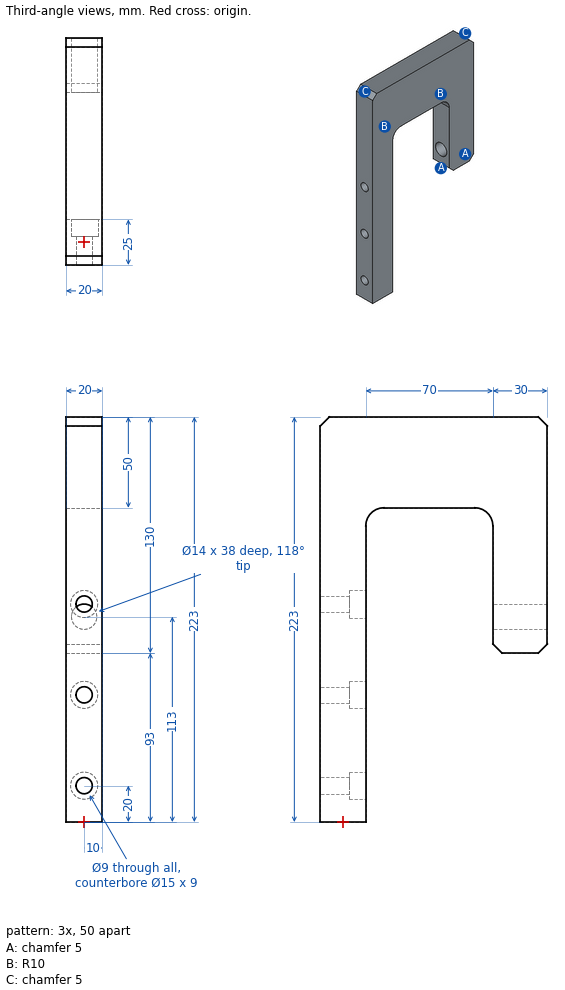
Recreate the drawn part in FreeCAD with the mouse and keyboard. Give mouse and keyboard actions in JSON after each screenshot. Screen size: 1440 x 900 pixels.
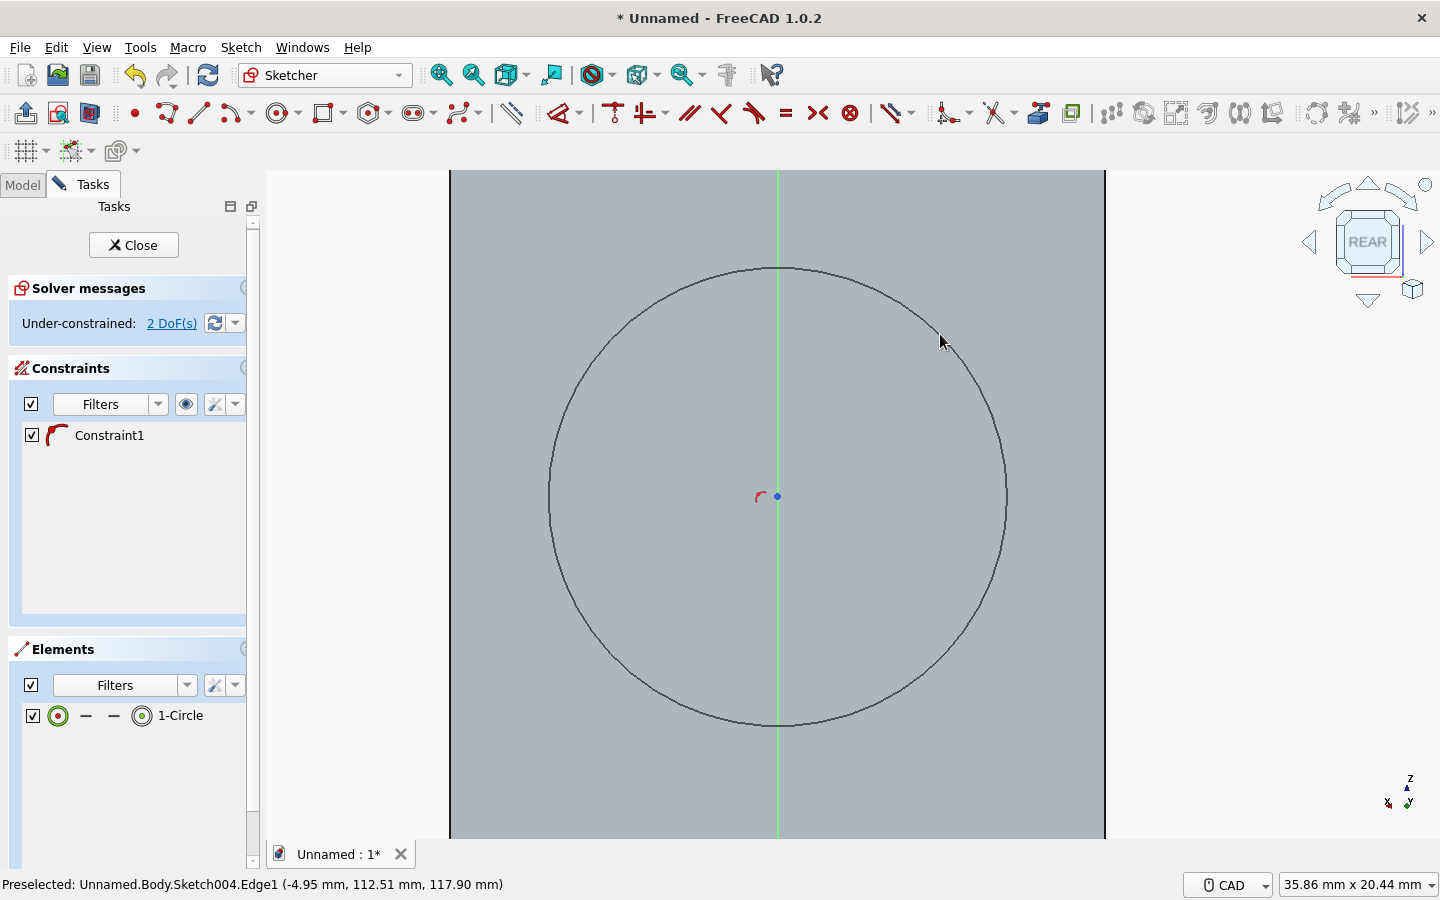
{"action": "left_click", "coordinate": [558, 114]}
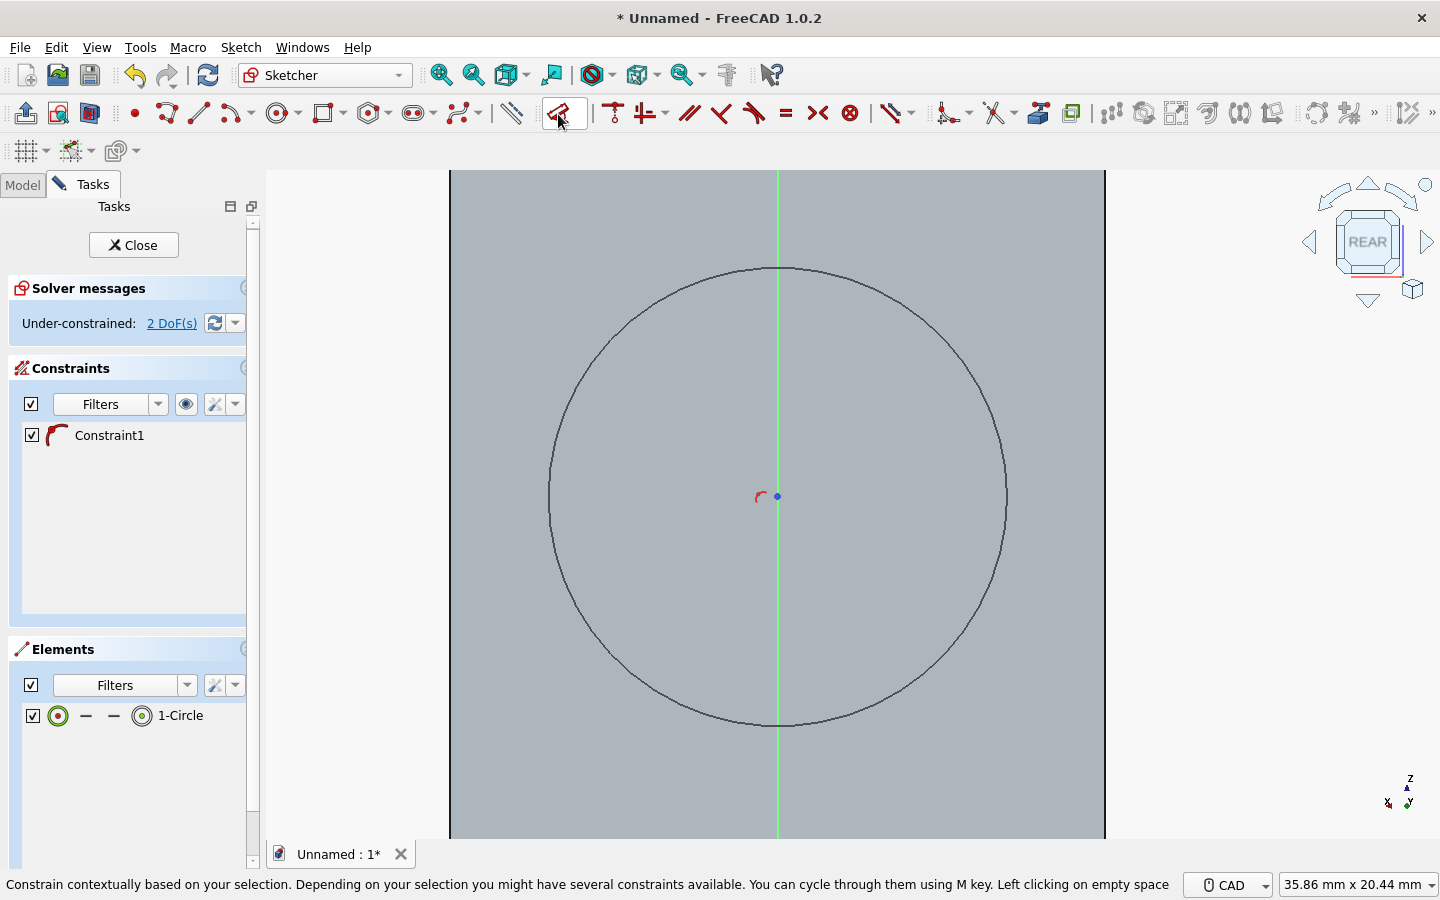
{"action": "left_click", "coordinate": [939, 334]}
{"action": "left_click", "coordinate": [962, 311]}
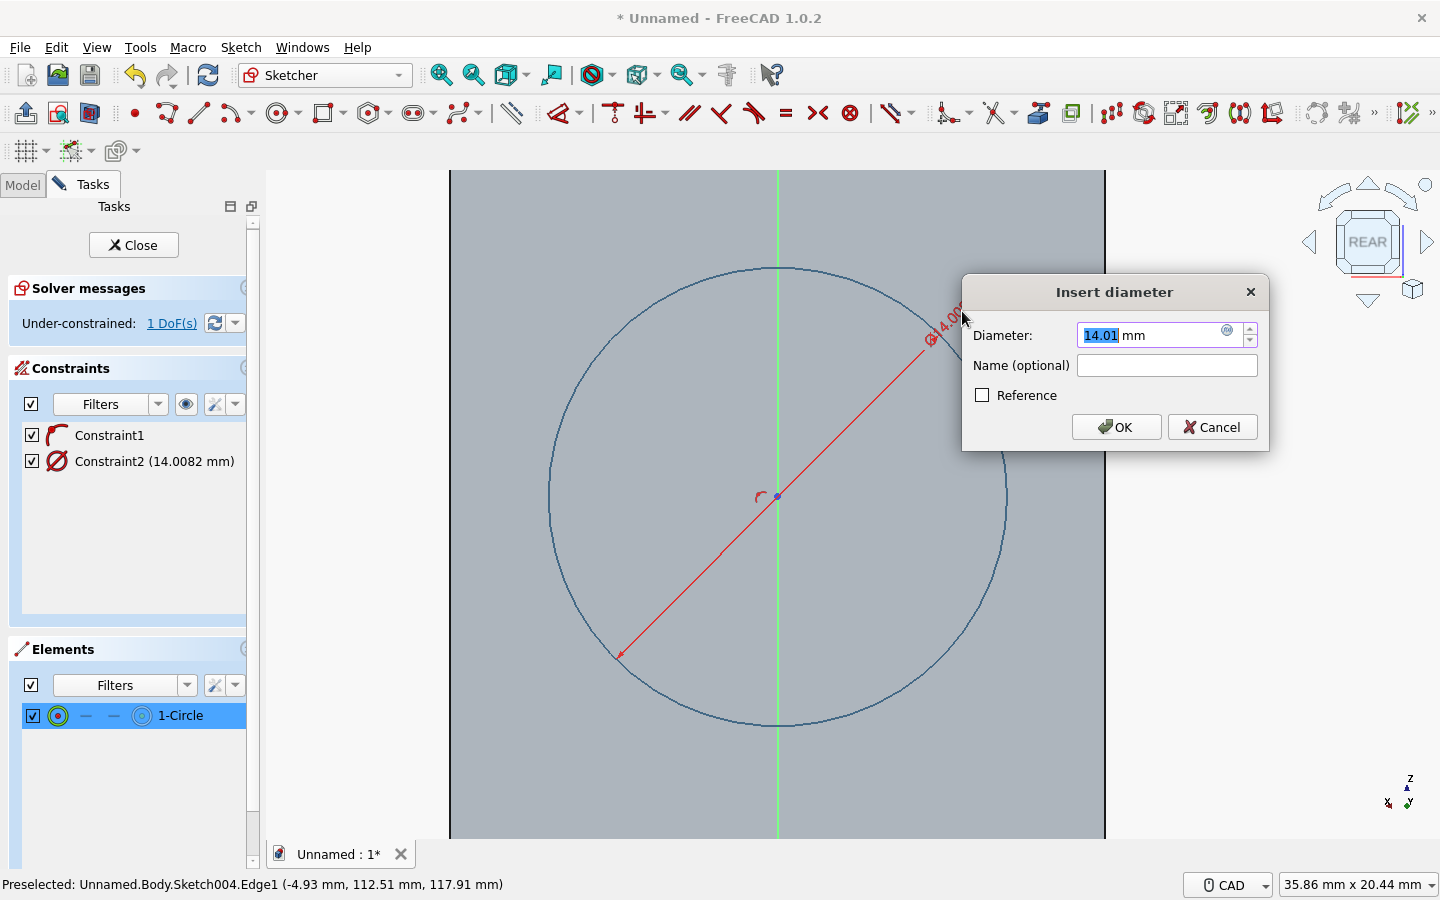
{"action": "type", "text": "14"}
{"action": "key", "text": "Return"}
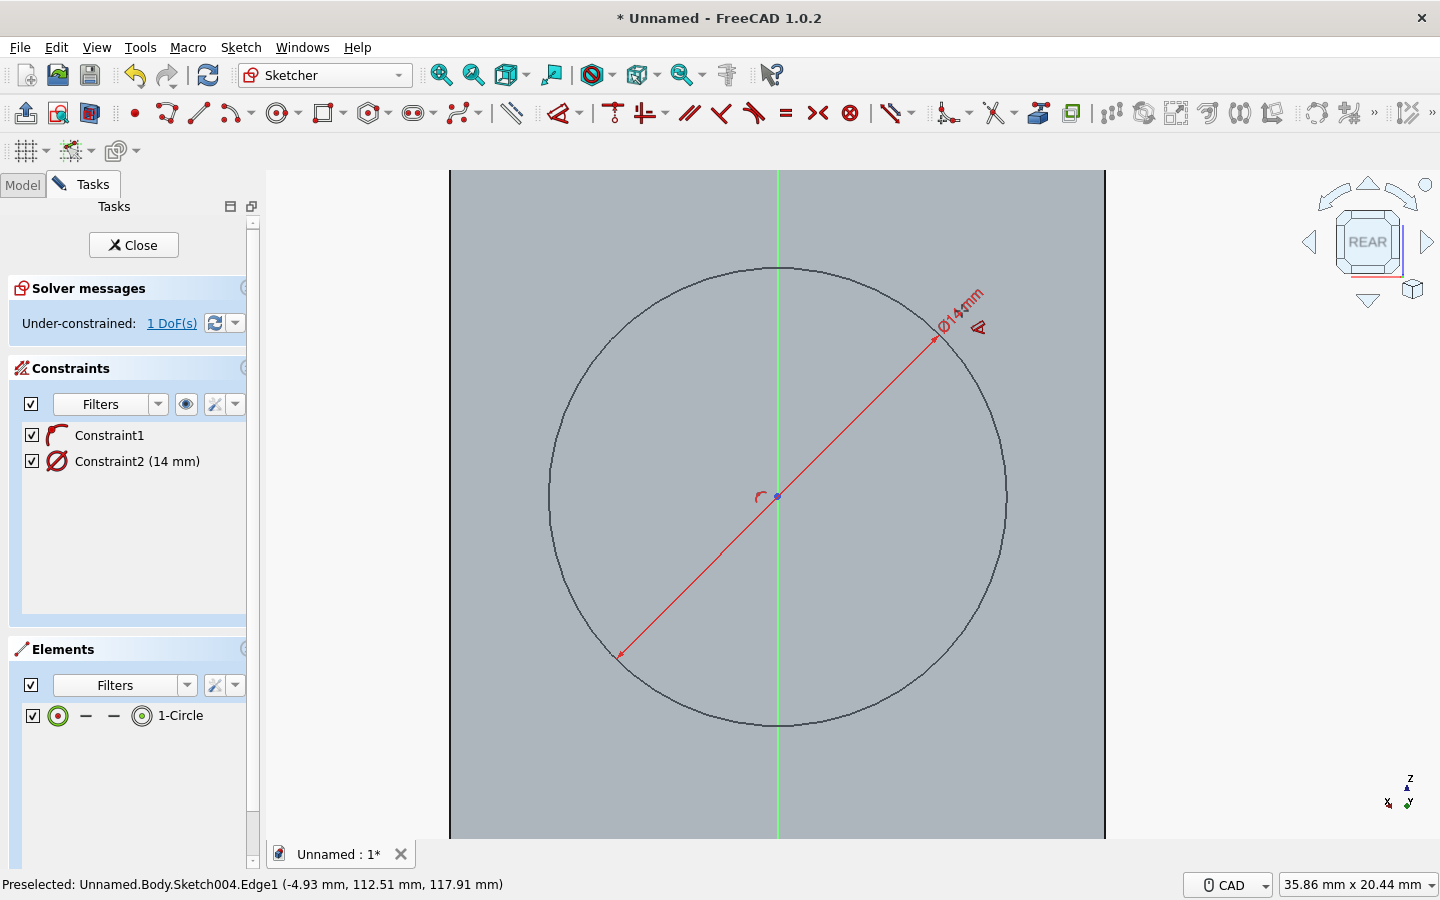
{"action": "left_click", "coordinate": [778, 497]}
{"action": "left_click", "coordinate": [812, 654]}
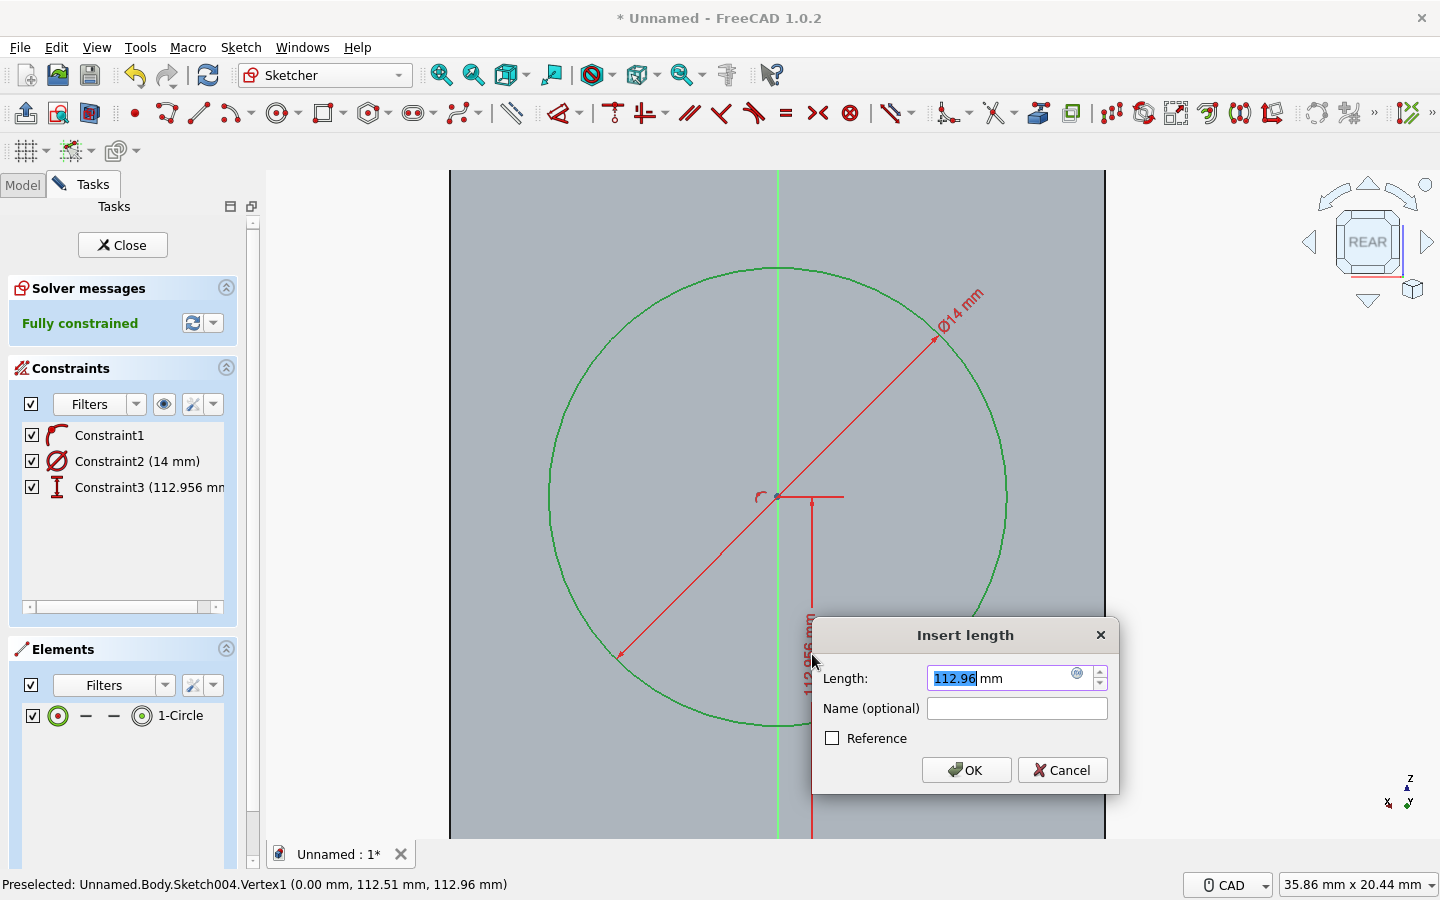
{"action": "type", "text": "113"}
{"action": "key", "text": "Return"}
{"action": "key", "text": "Escape"}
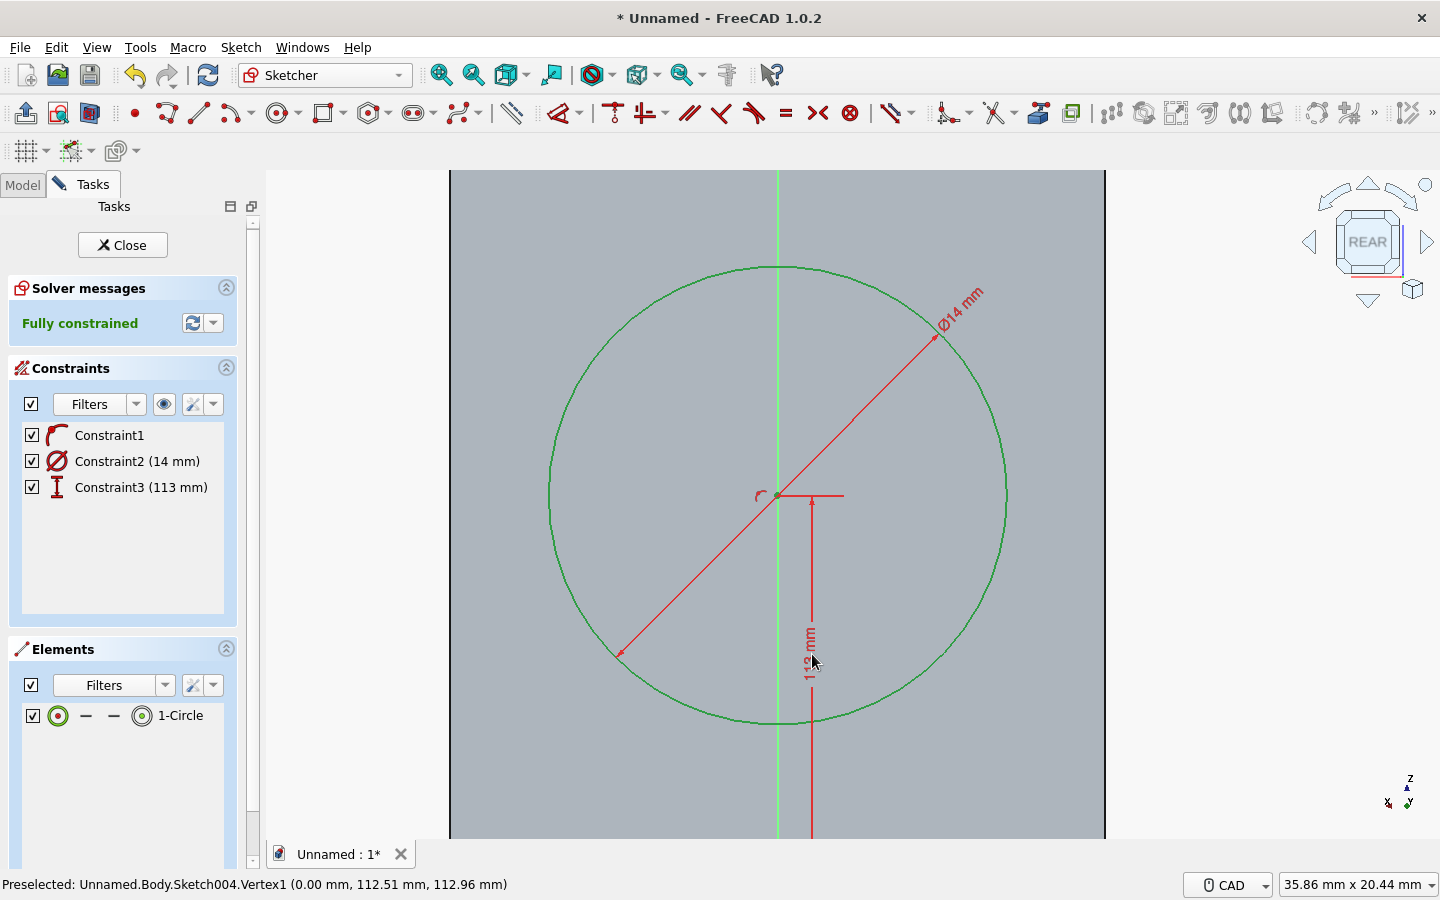
{"action": "left_click", "coordinate": [123, 245]}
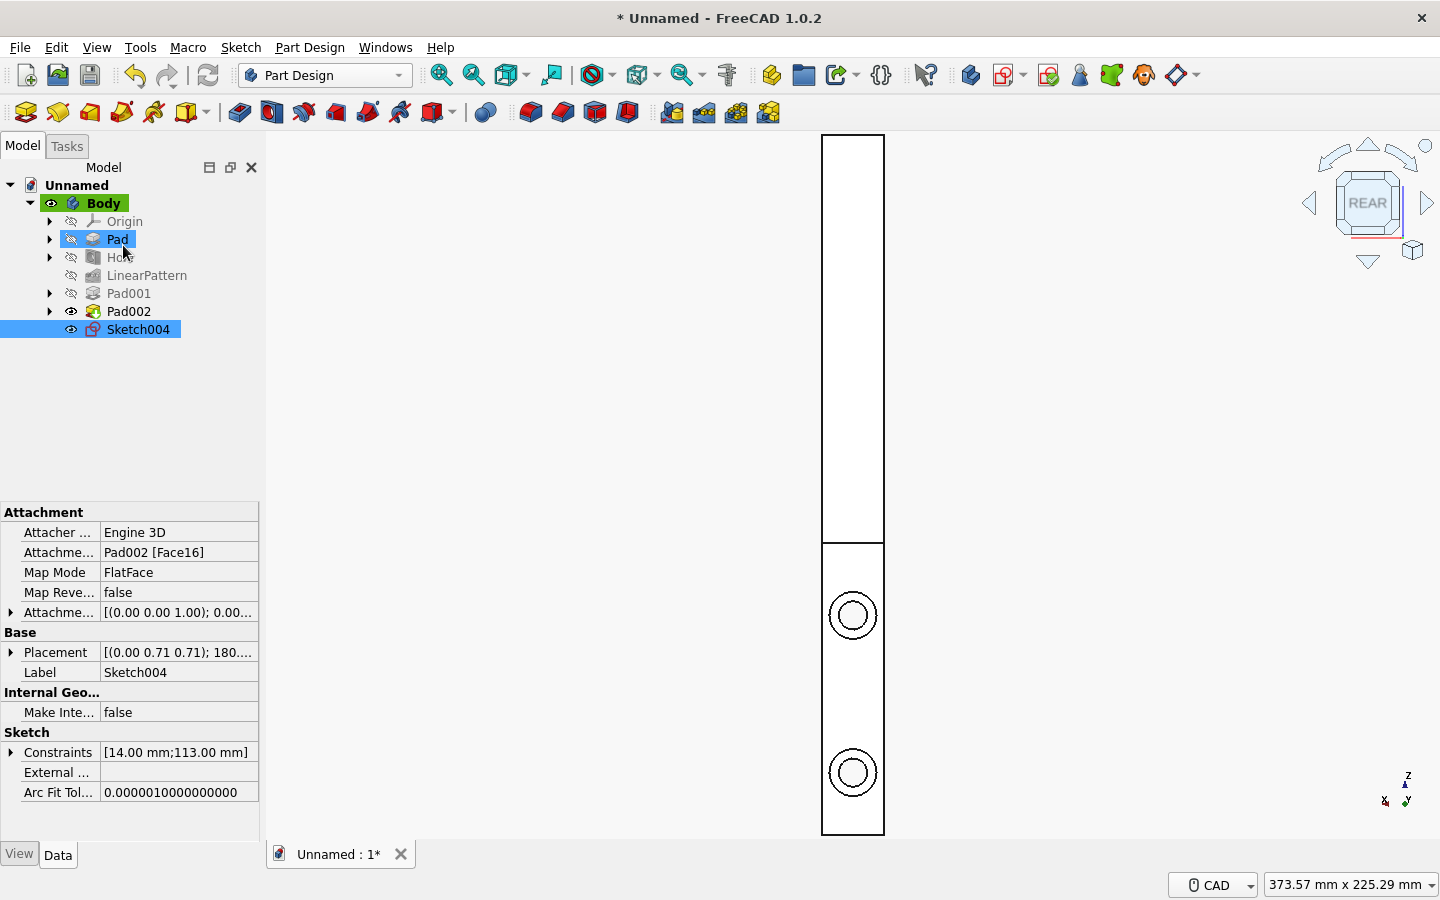
{"action": "left_click", "coordinate": [272, 112]}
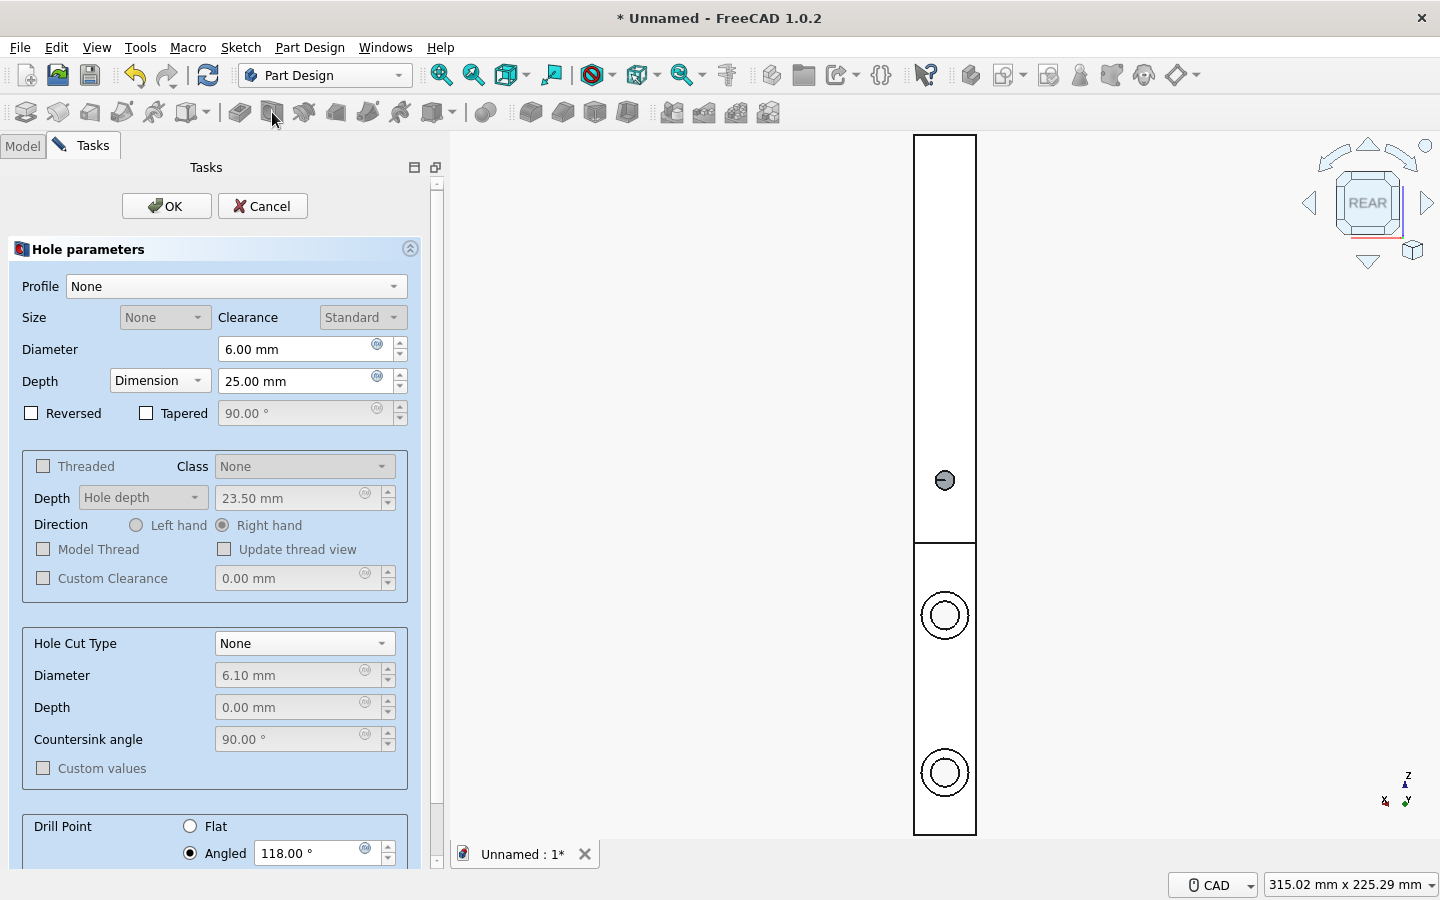
{"action": "triple_click", "coordinate": [305, 349]}